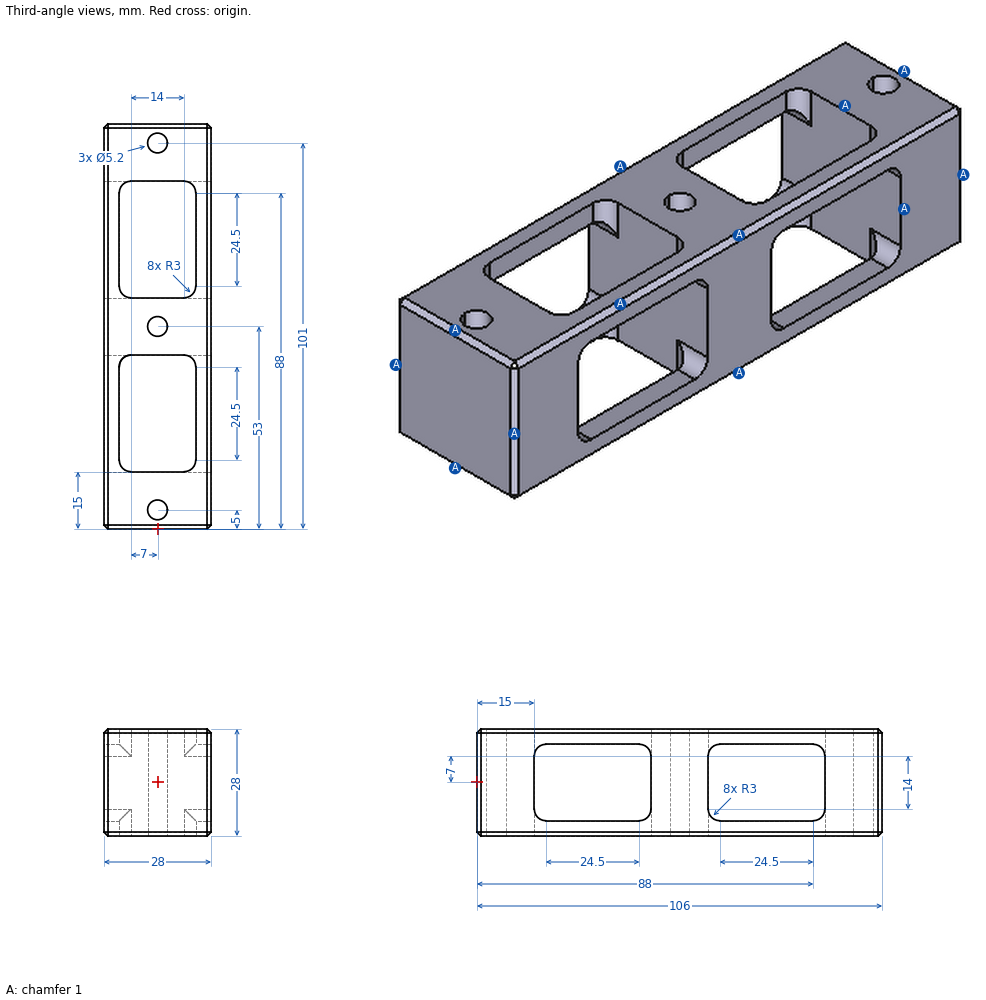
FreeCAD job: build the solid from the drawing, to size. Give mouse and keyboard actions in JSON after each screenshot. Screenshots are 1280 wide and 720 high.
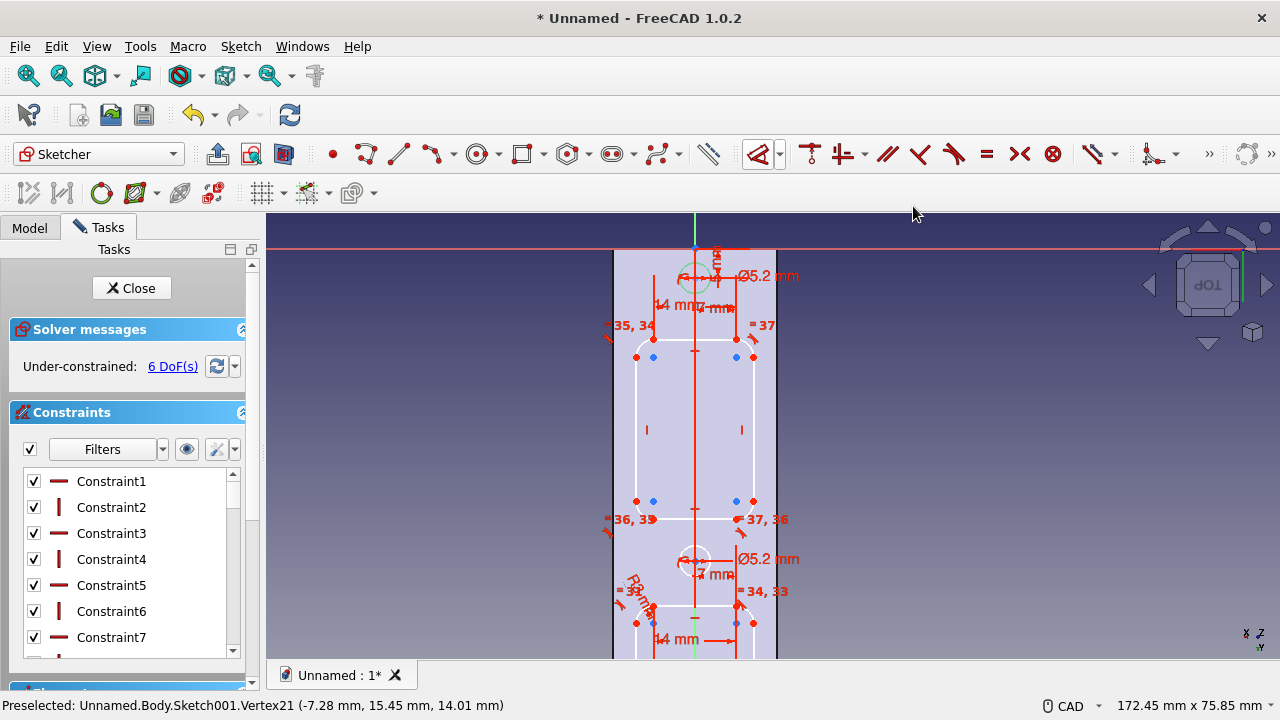
{"action": "left_click", "coordinate": [695, 561]}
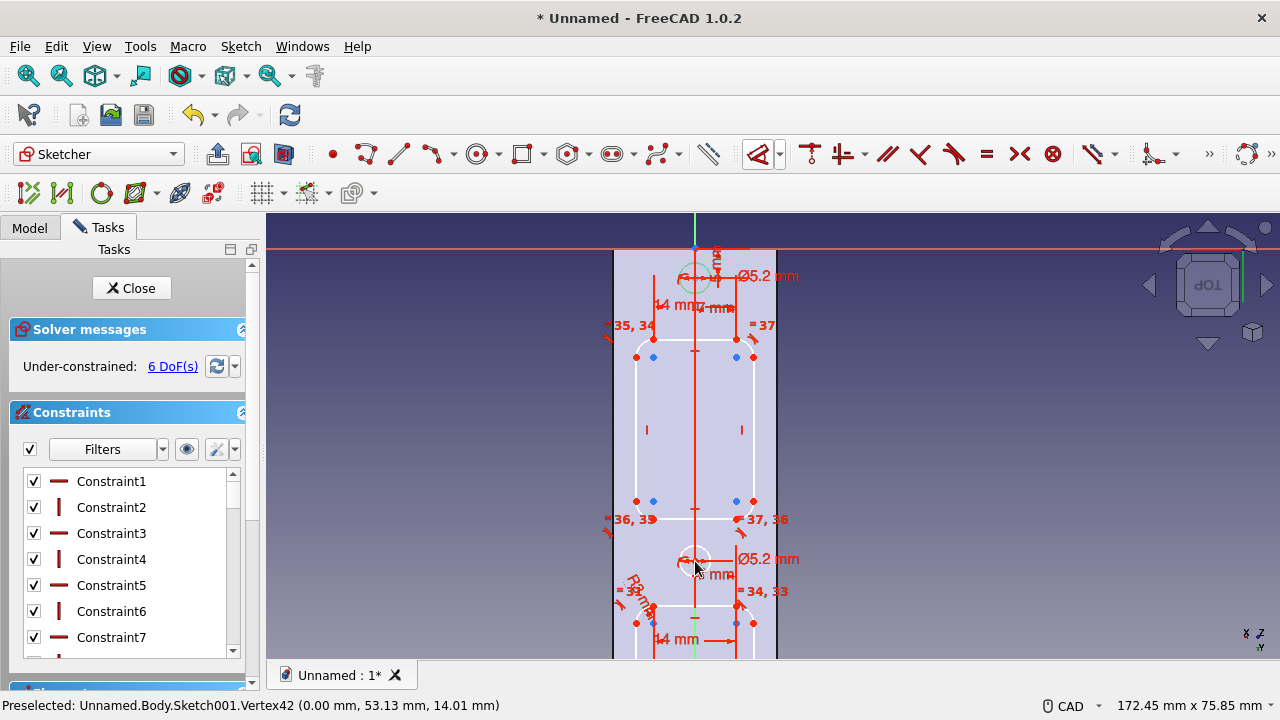
{"action": "key", "text": "i"}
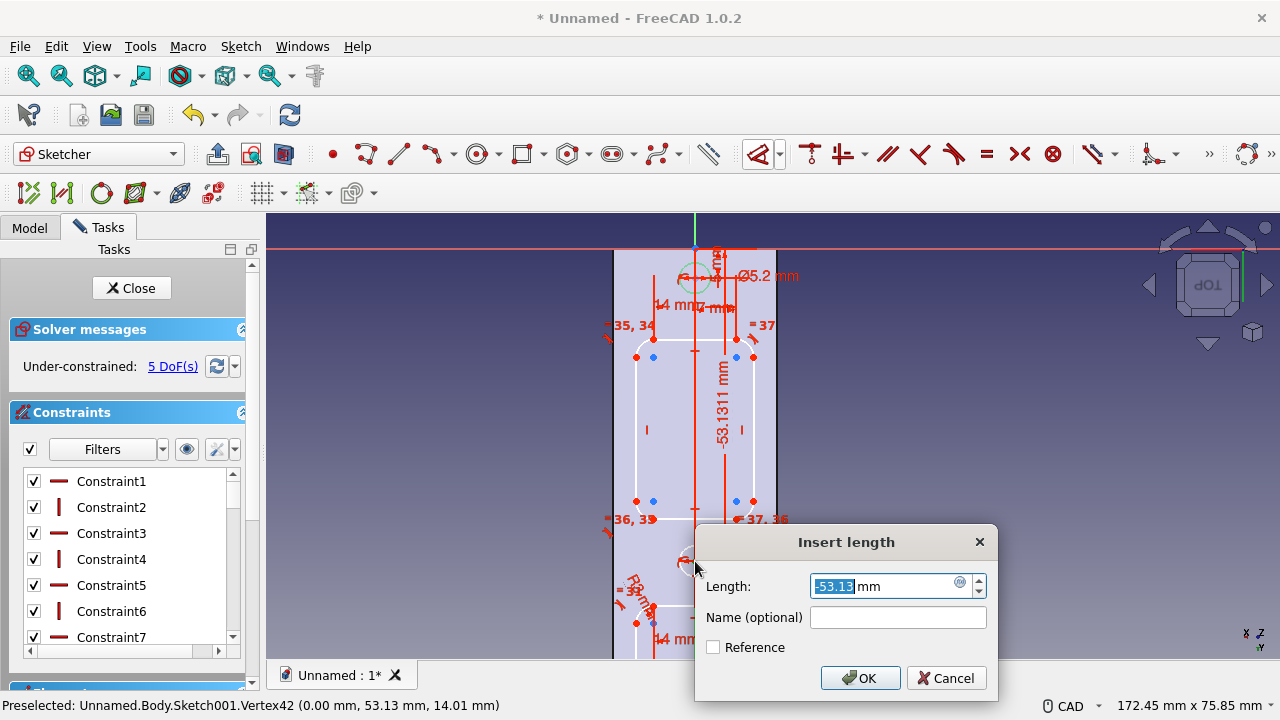
{"action": "type", "text": "-53"}
{"action": "key", "text": "Return"}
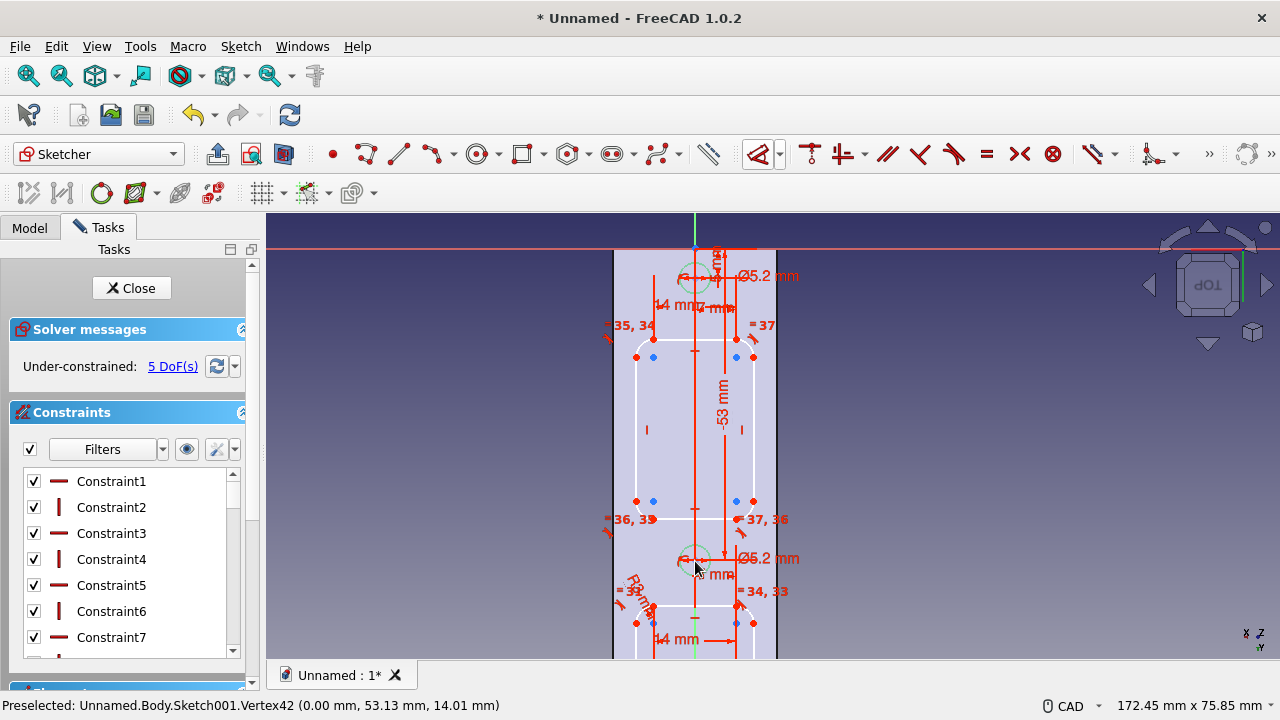
{"action": "scroll", "coordinate": [712, 340], "scroll_direction": "down", "scroll_amount": 4}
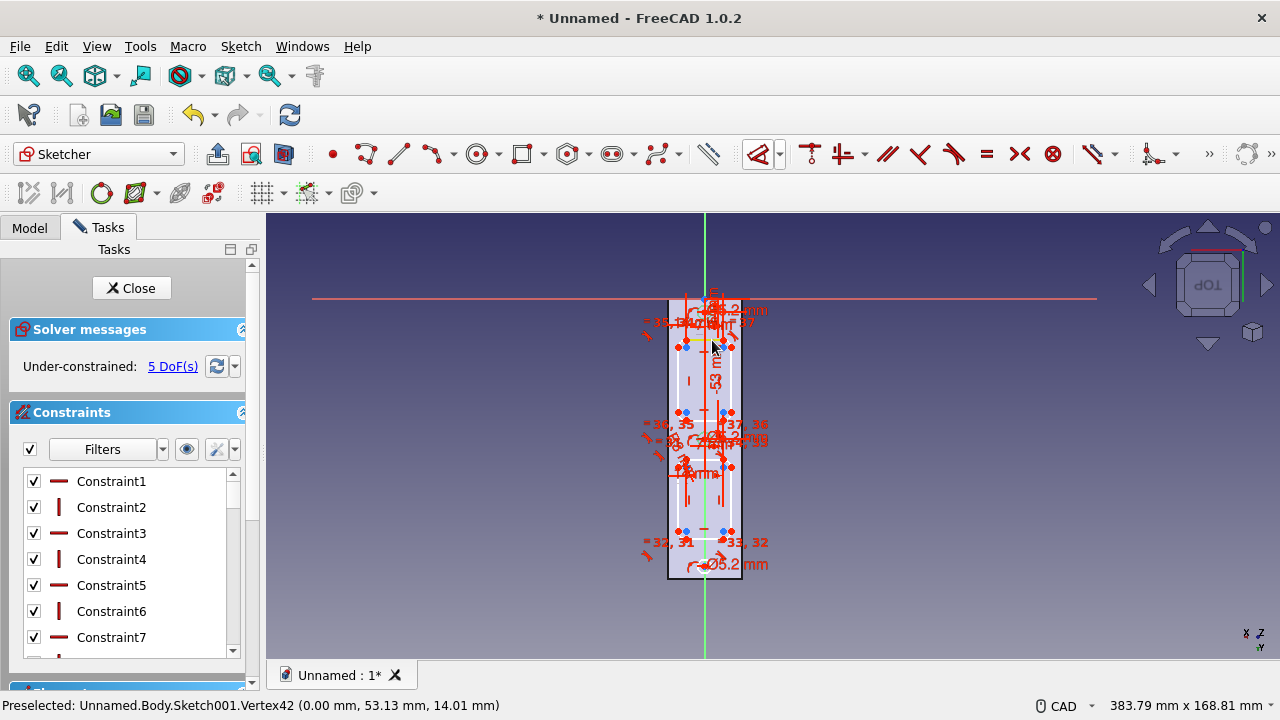
{"action": "scroll", "coordinate": [678, 531], "scroll_direction": "up", "scroll_amount": 3}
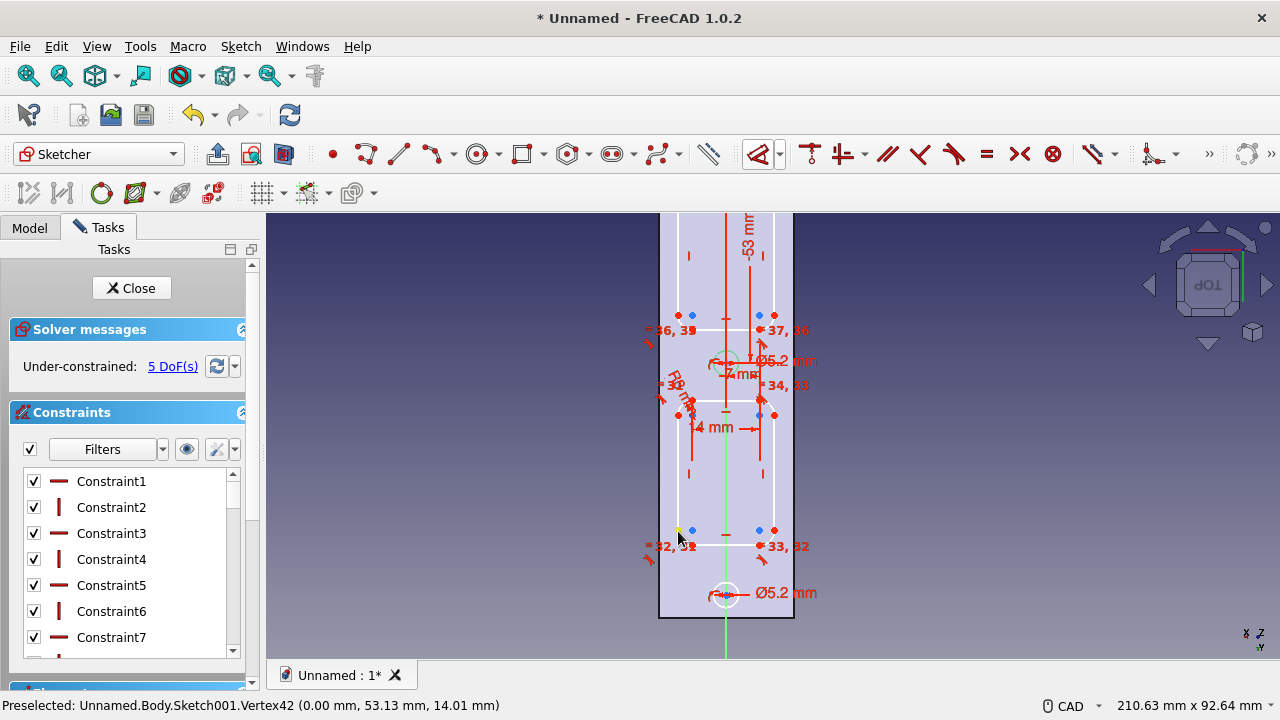
{"action": "left_click", "coordinate": [678, 531]}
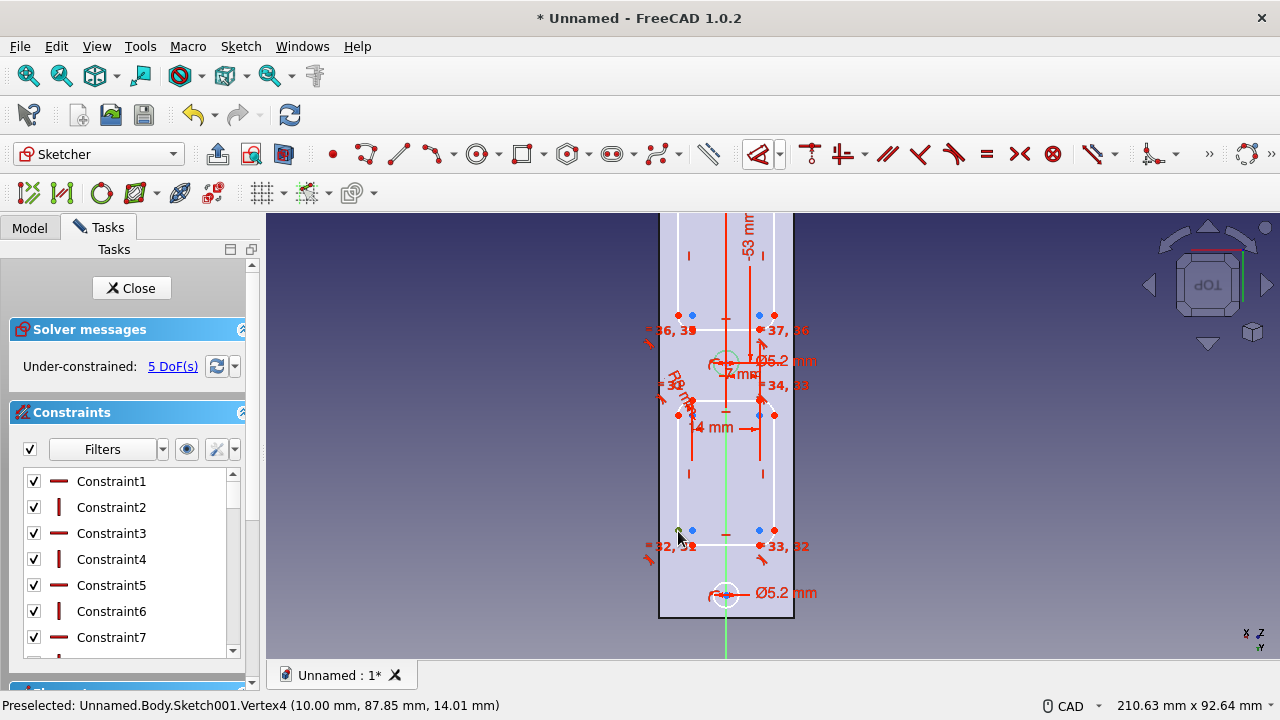
{"action": "key", "text": "i"}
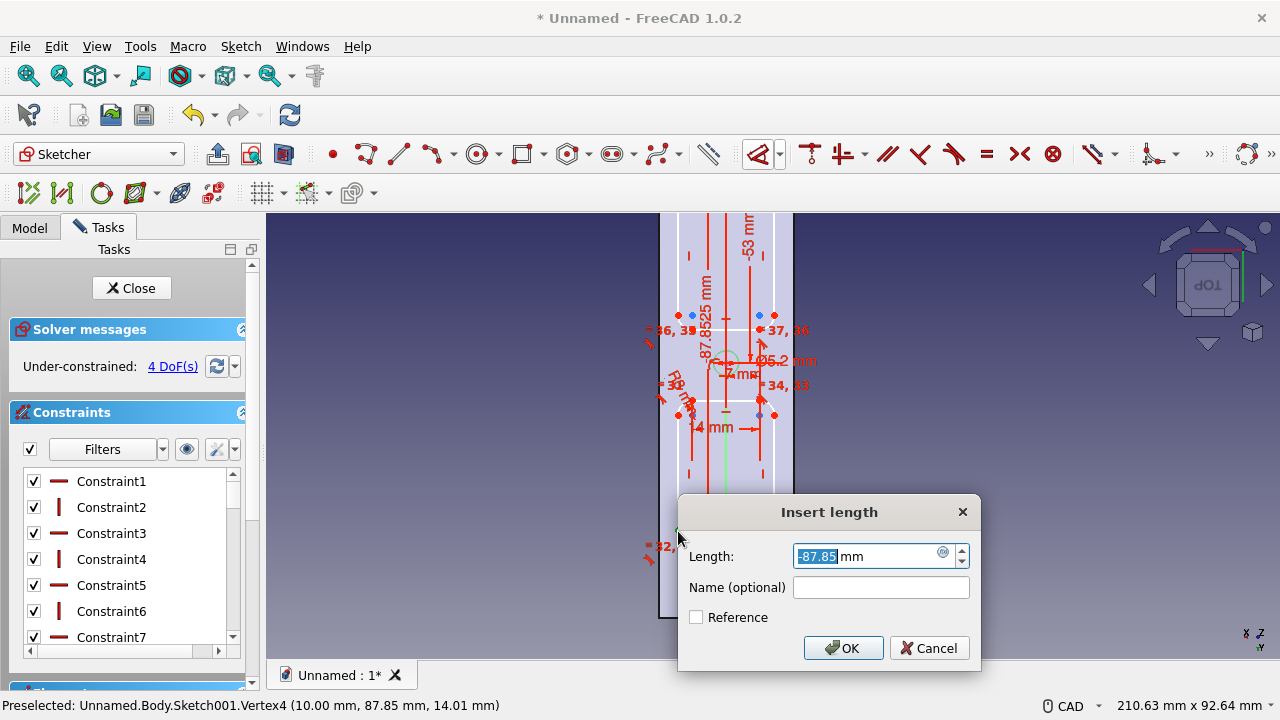
{"action": "type", "text": "-88"}
{"action": "key", "text": "Return"}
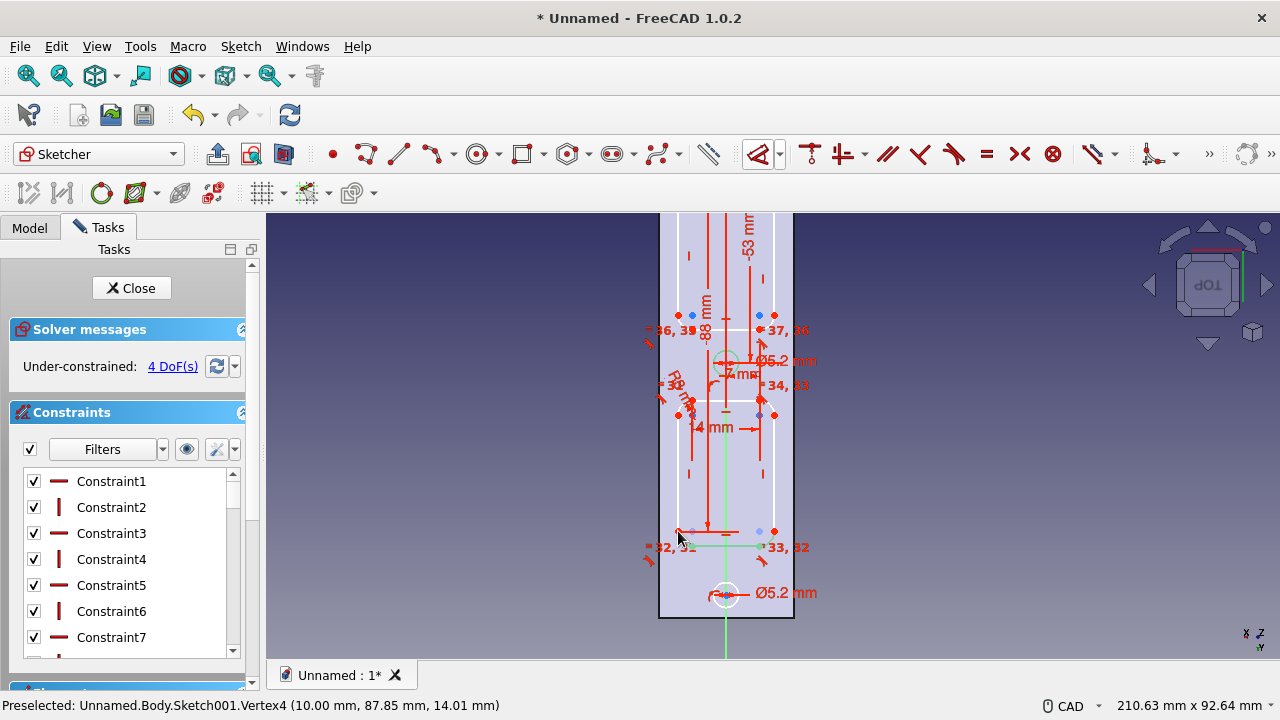
{"action": "scroll", "coordinate": [678, 532], "scroll_direction": "down", "scroll_amount": 3}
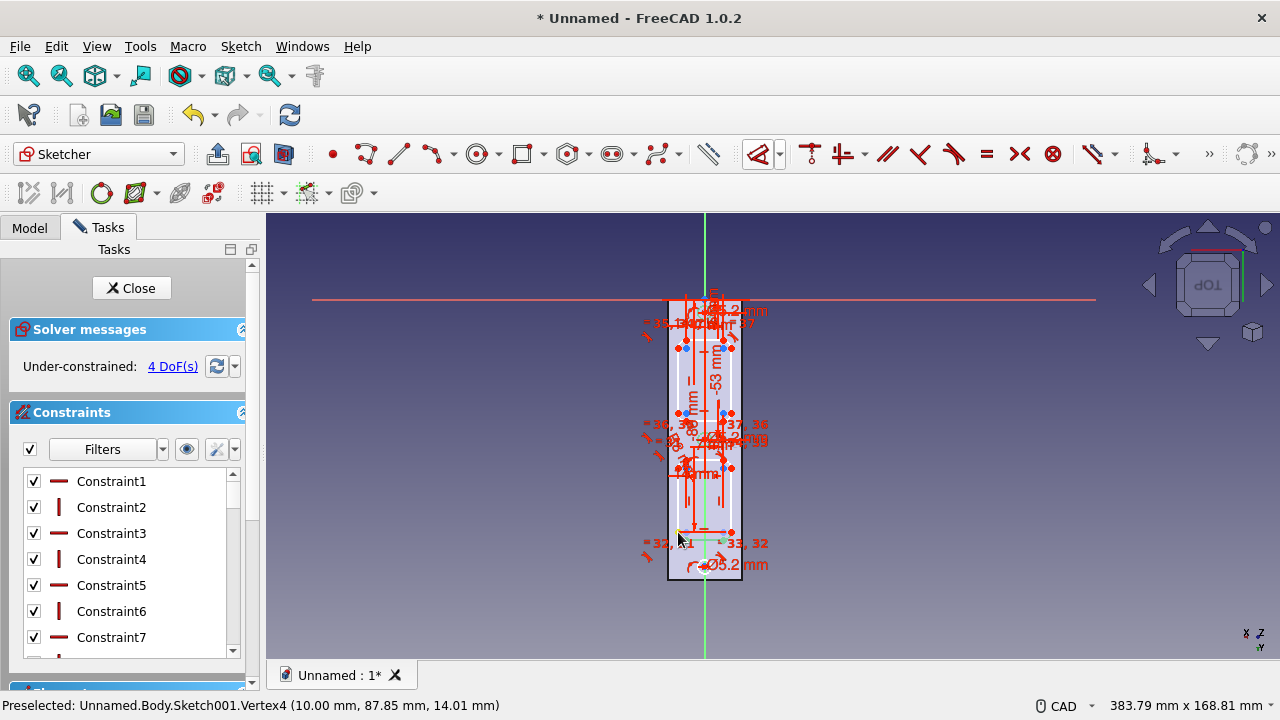
{"action": "scroll", "coordinate": [723, 340], "scroll_direction": "up", "scroll_amount": 3}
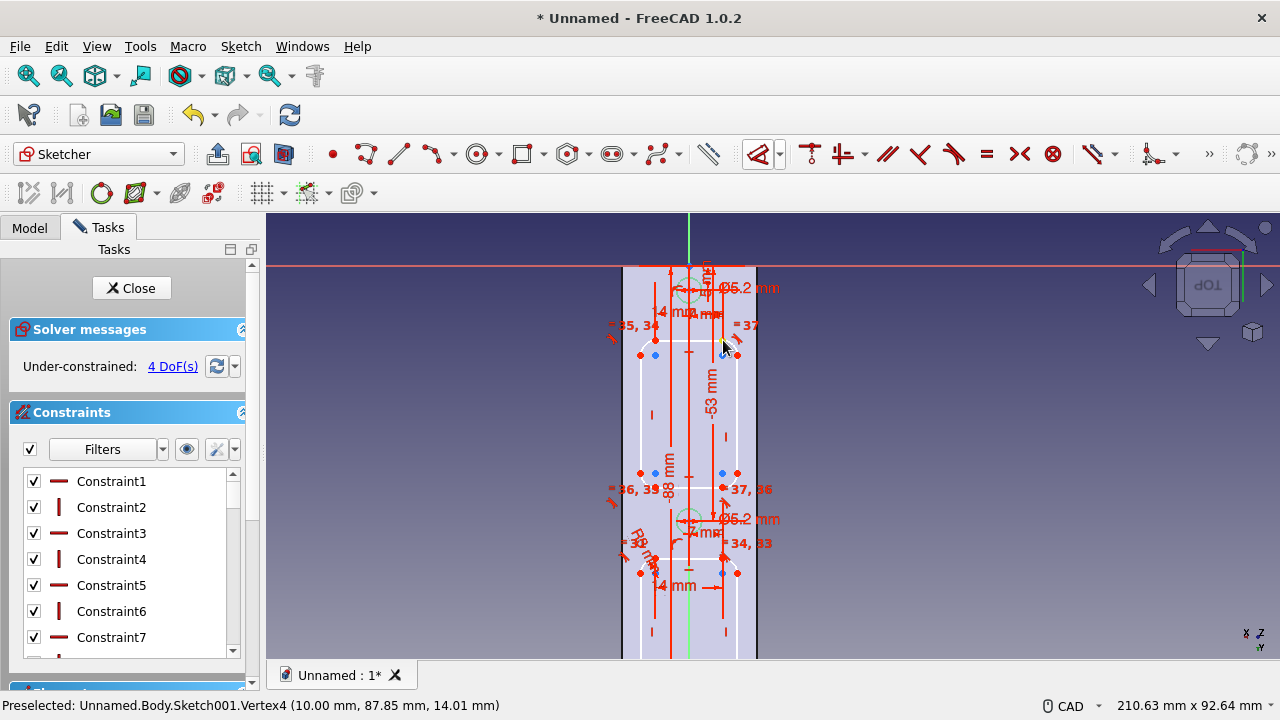
{"action": "left_click", "coordinate": [723, 341]}